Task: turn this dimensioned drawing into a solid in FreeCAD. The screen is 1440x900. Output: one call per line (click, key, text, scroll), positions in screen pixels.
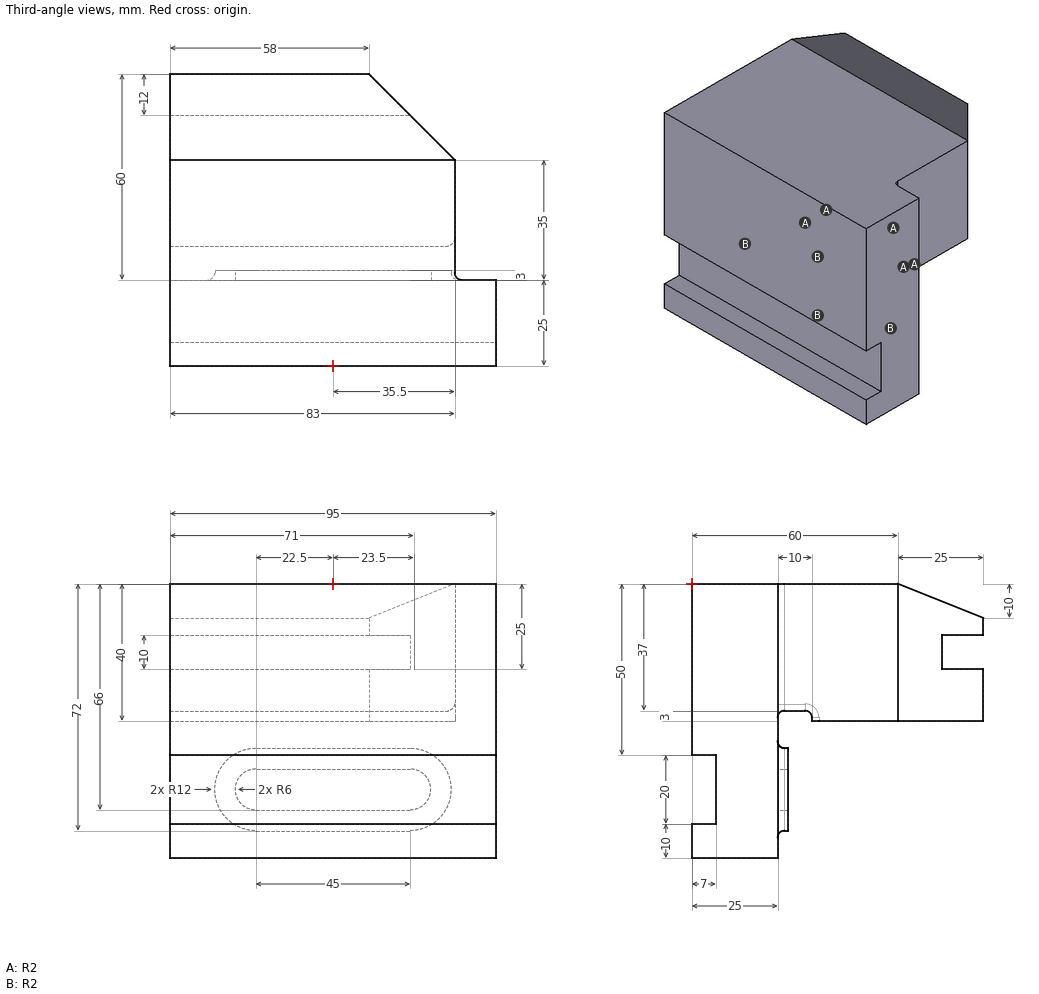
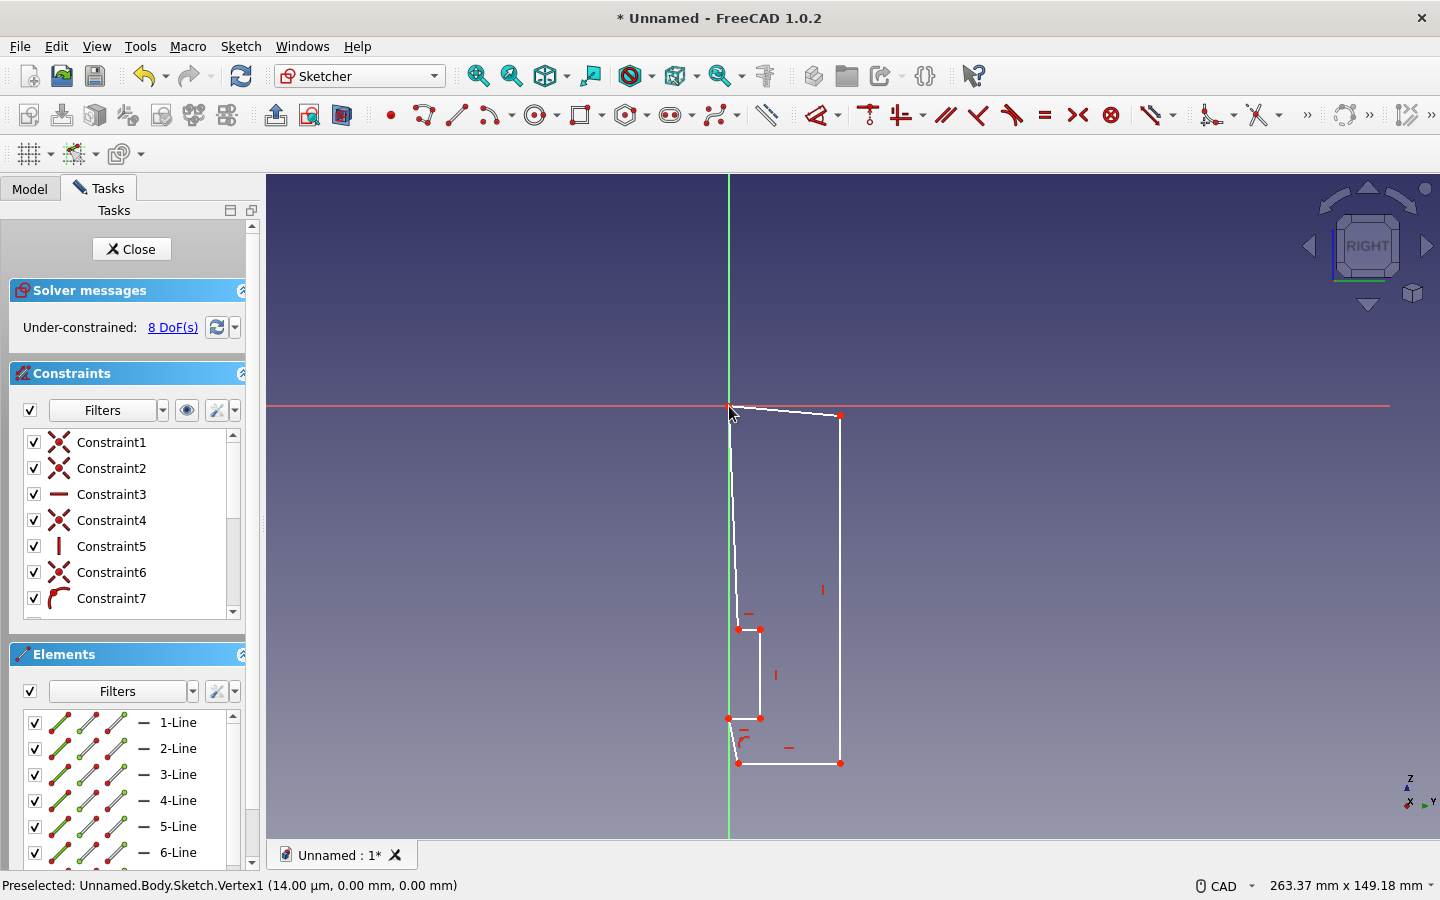
click(732, 473)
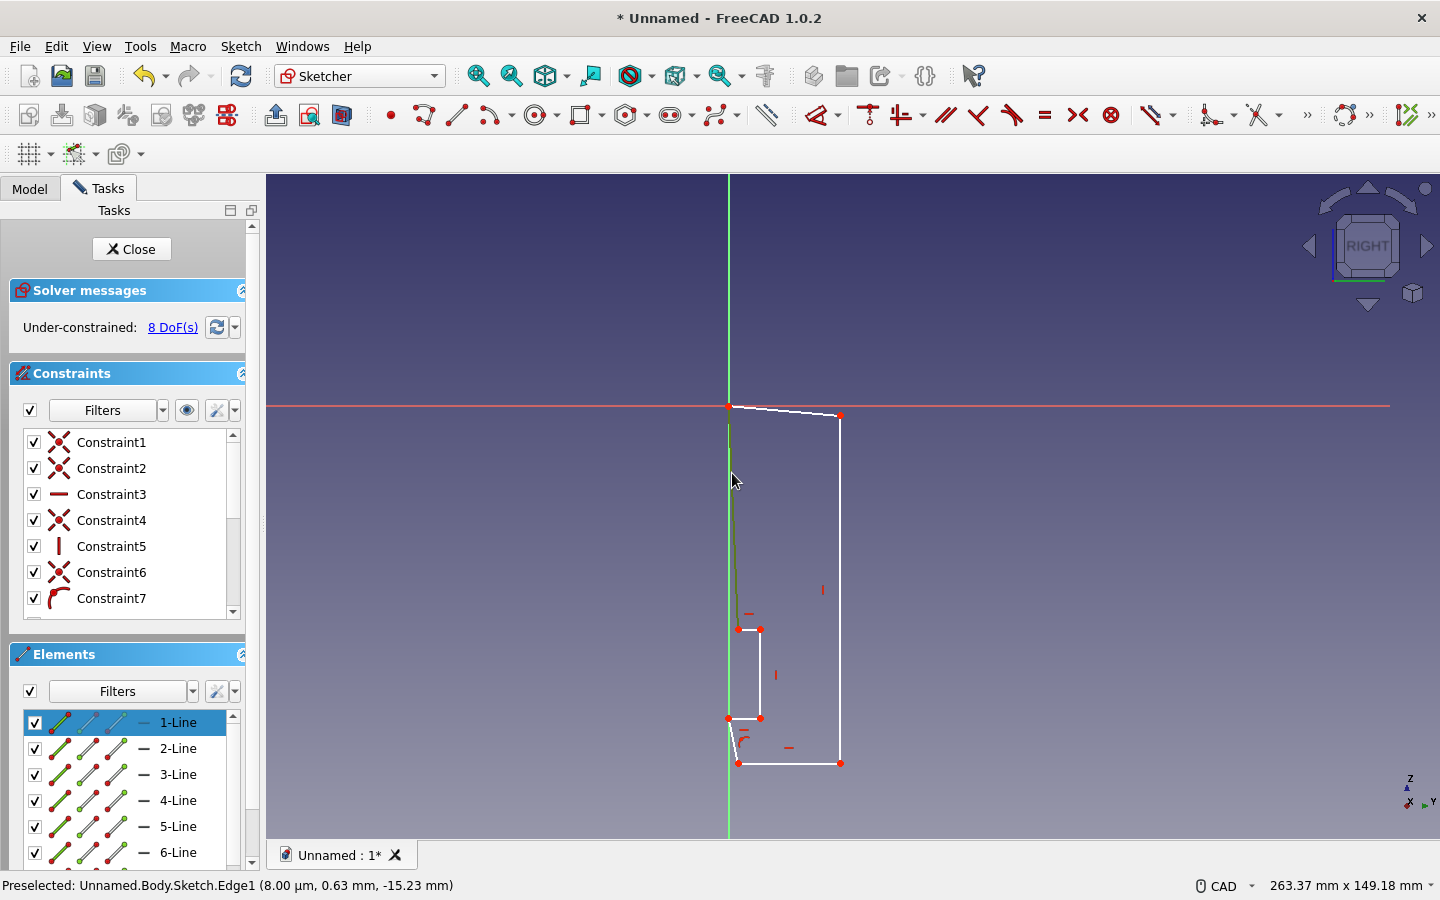
click(922, 116)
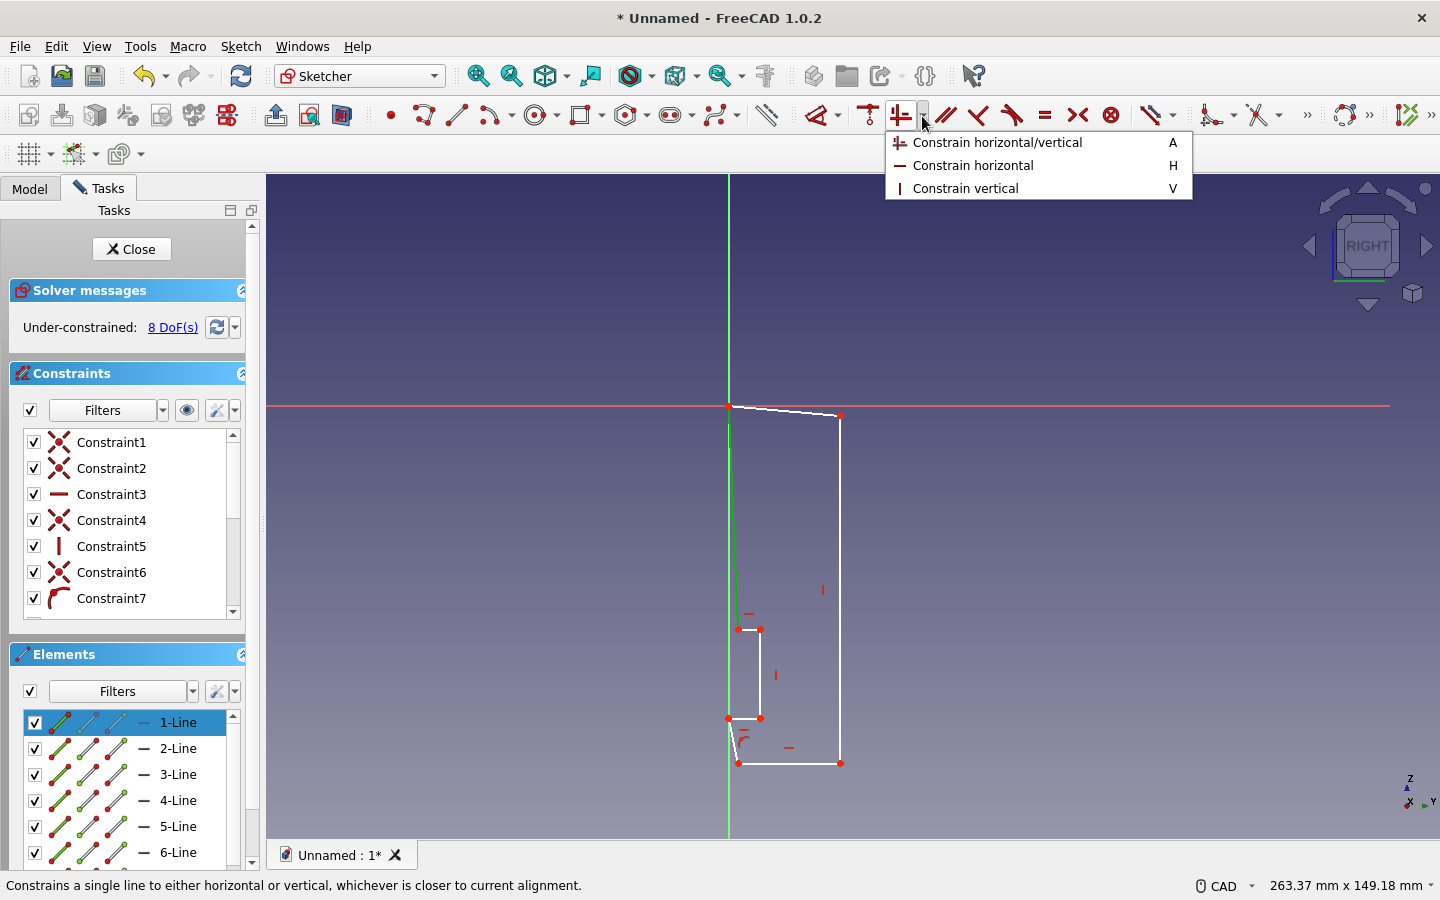
click(1039, 188)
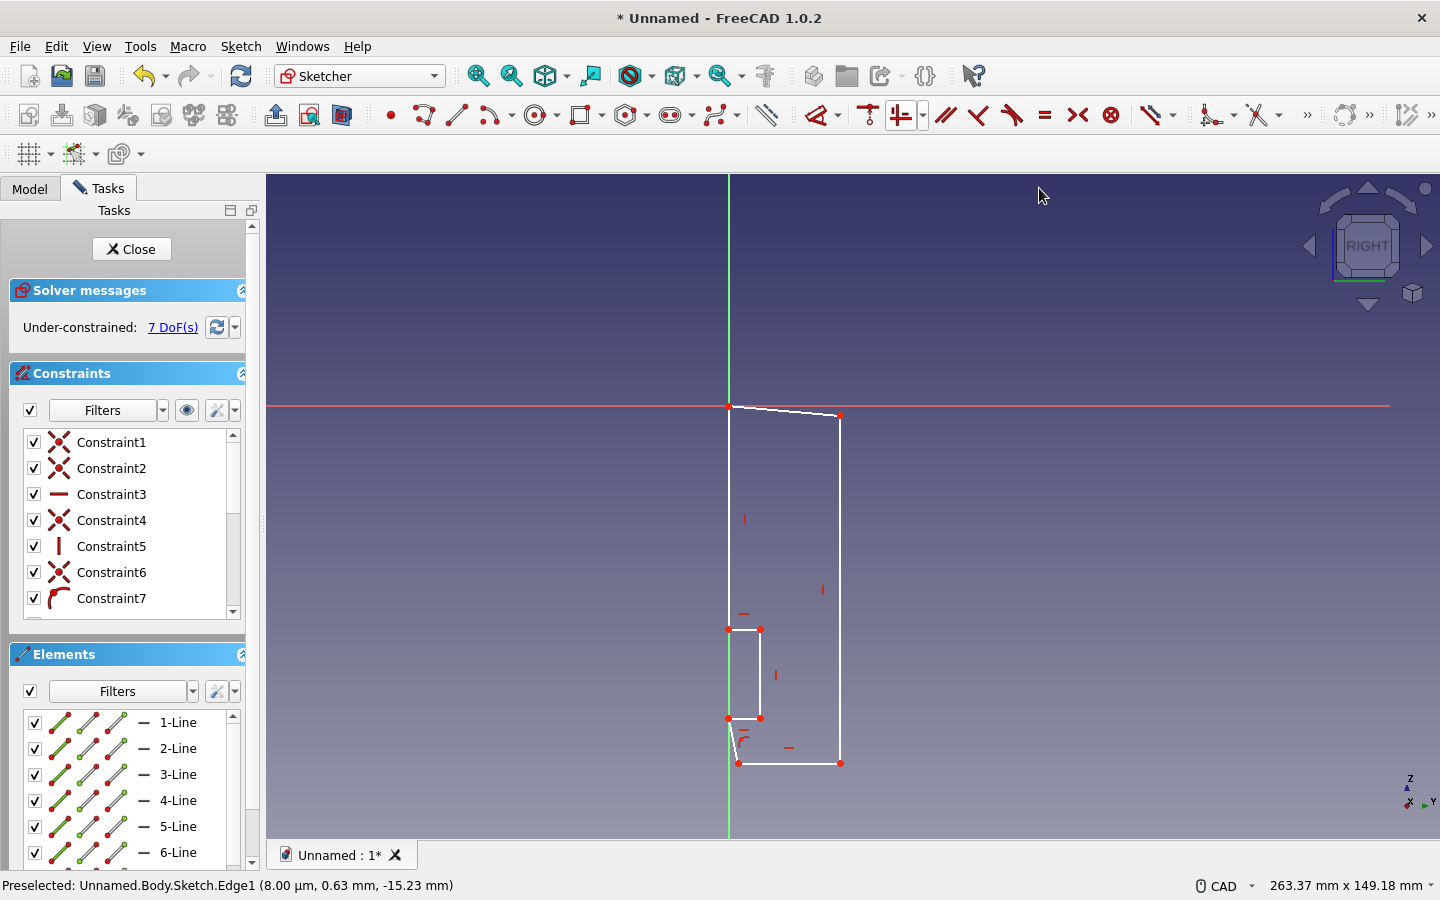
click(732, 732)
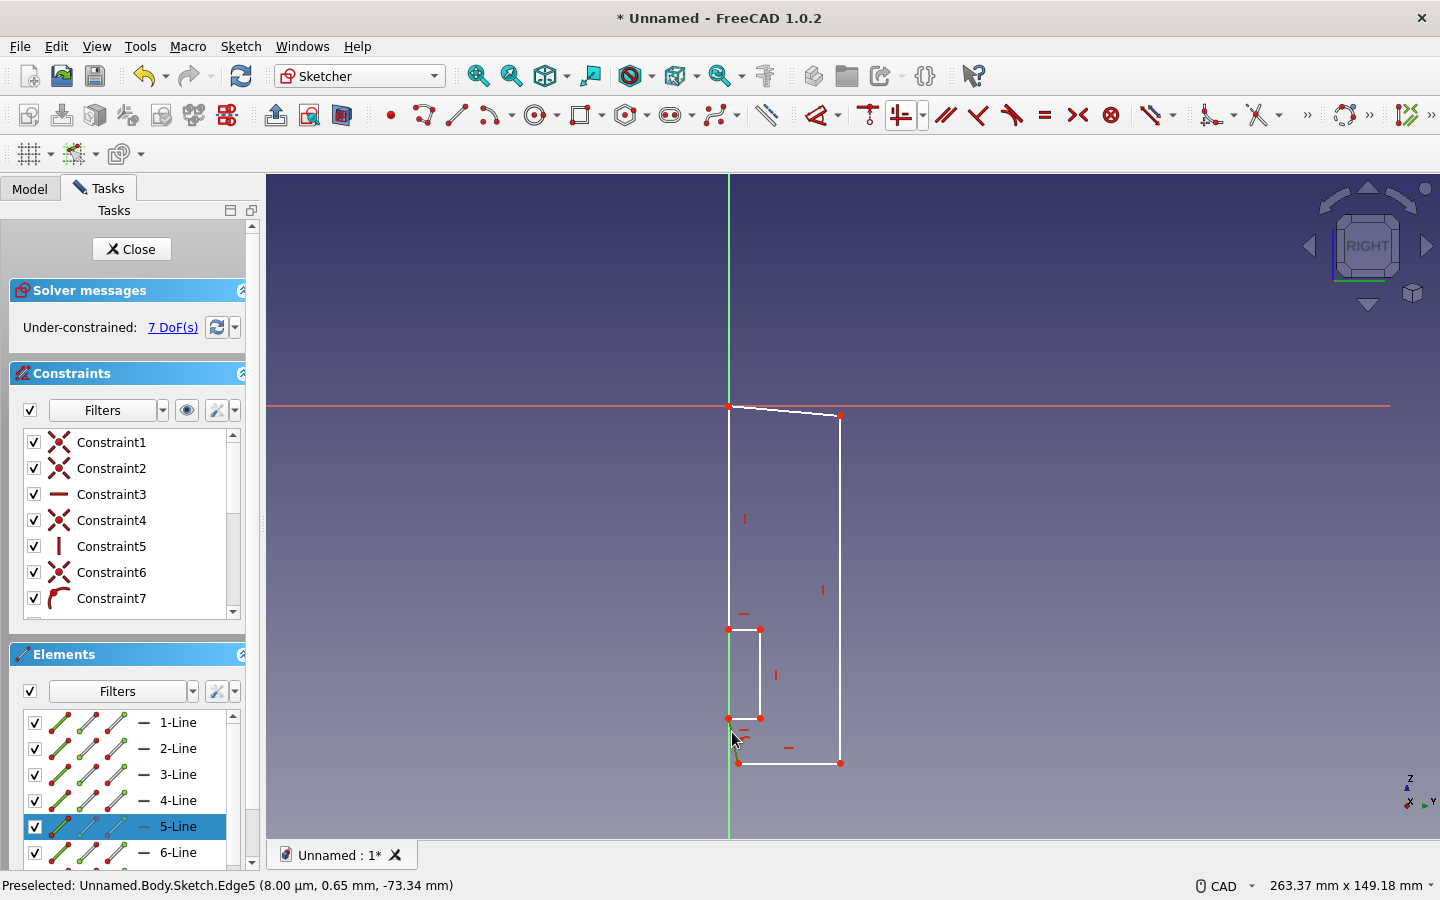
key(v)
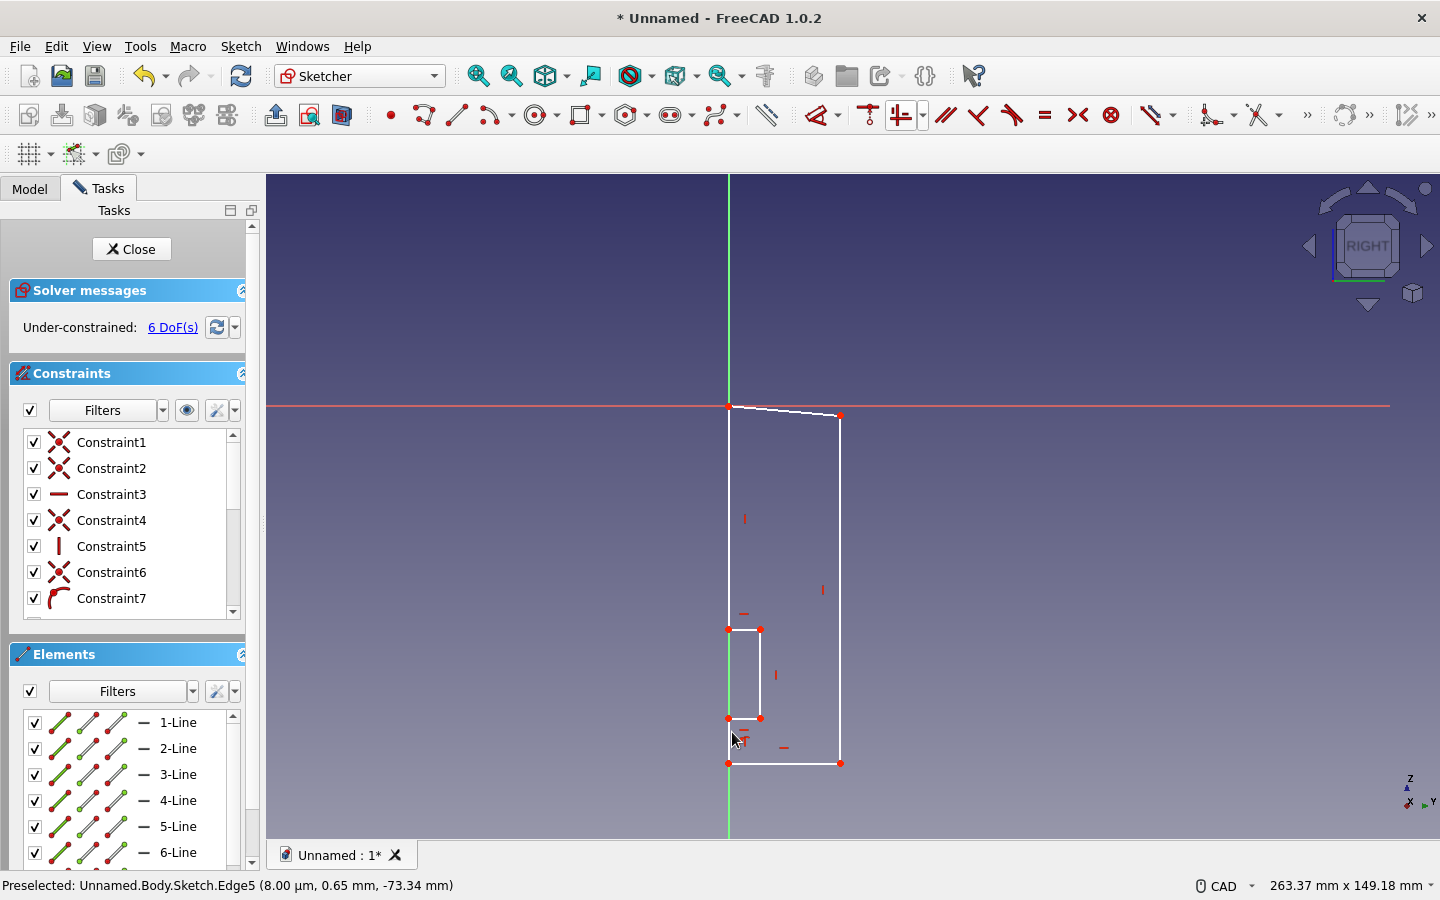
click(762, 409)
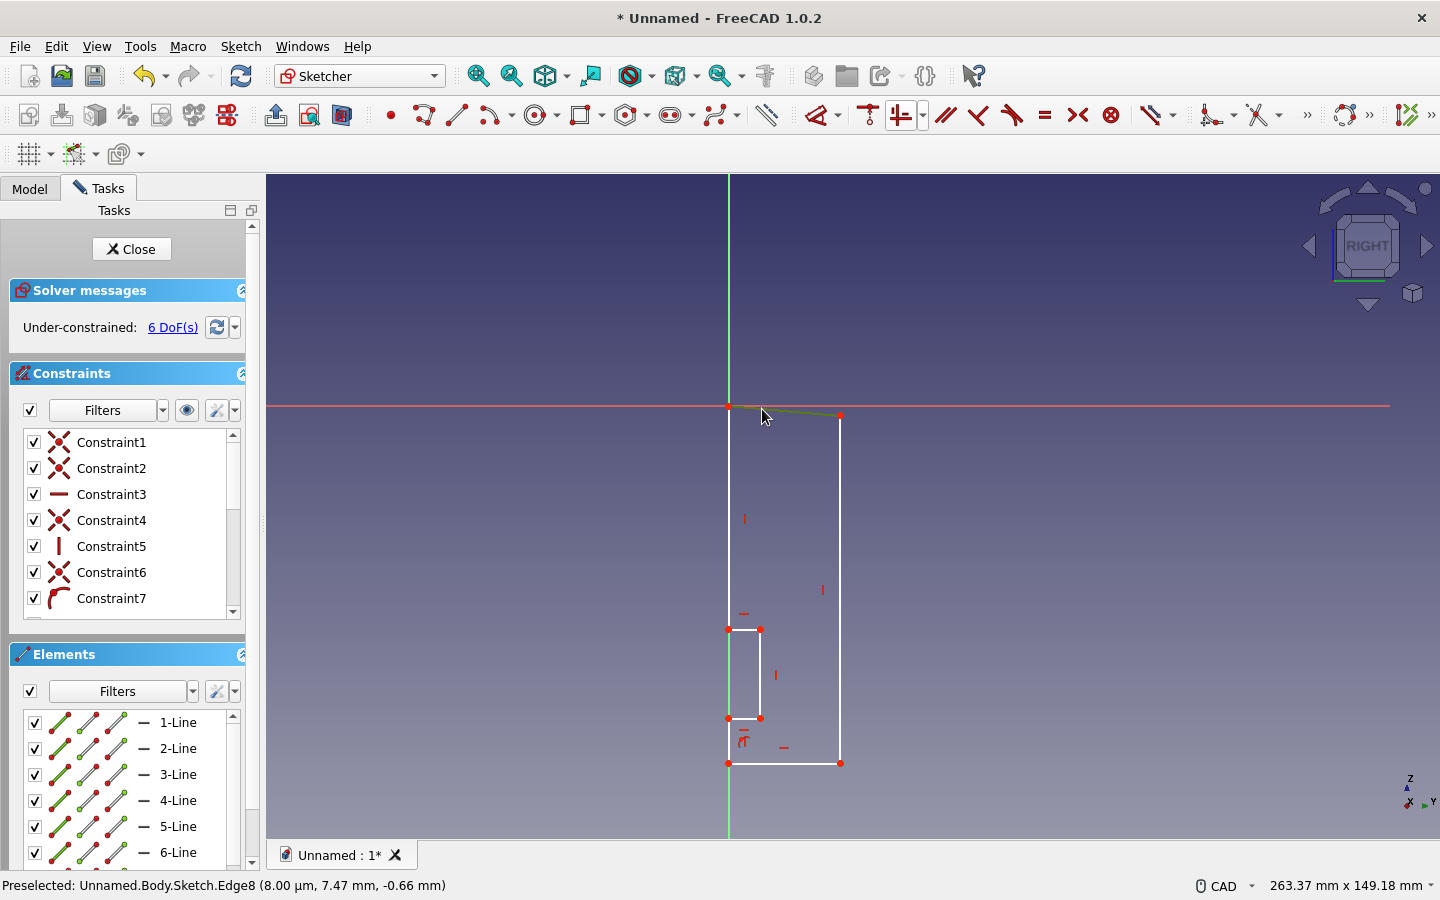
click(922, 116)